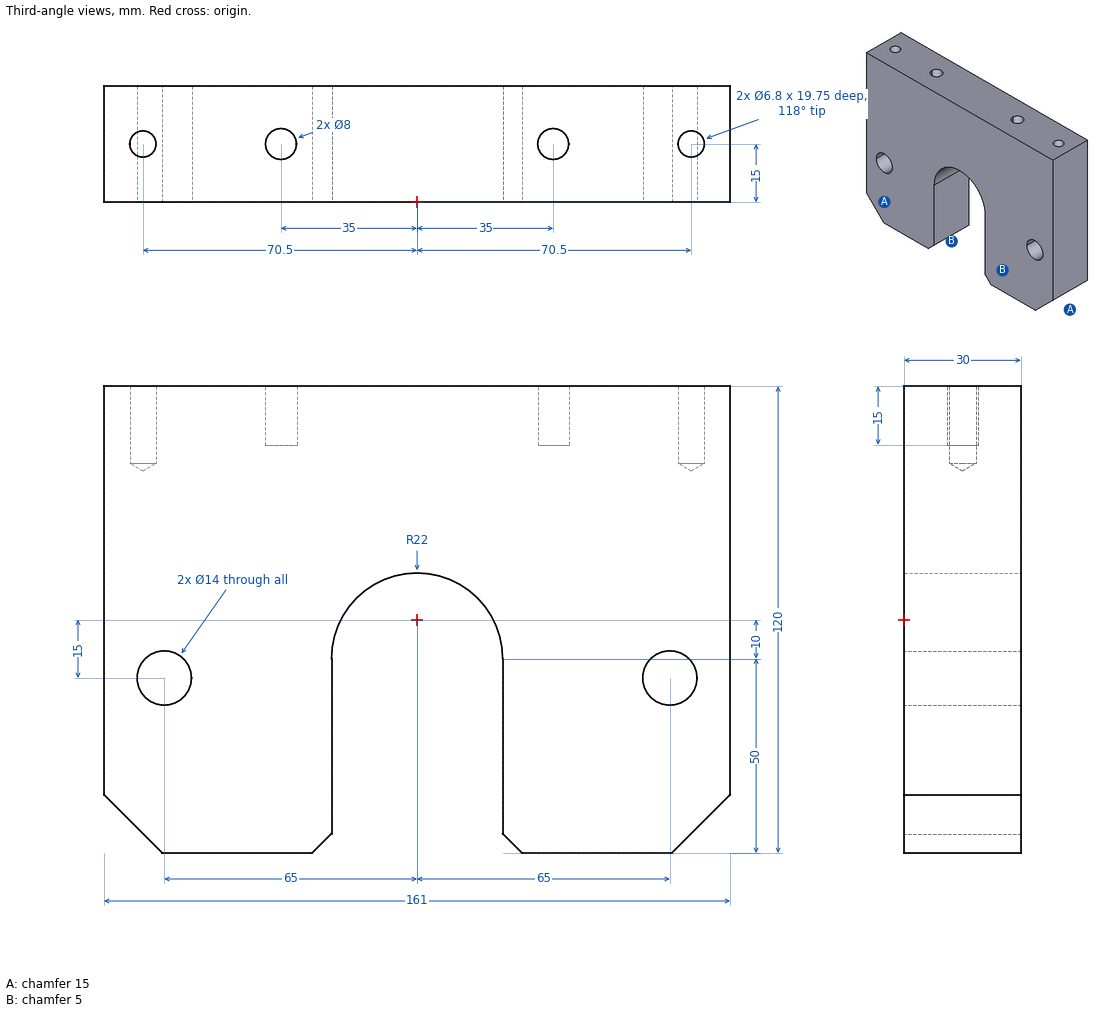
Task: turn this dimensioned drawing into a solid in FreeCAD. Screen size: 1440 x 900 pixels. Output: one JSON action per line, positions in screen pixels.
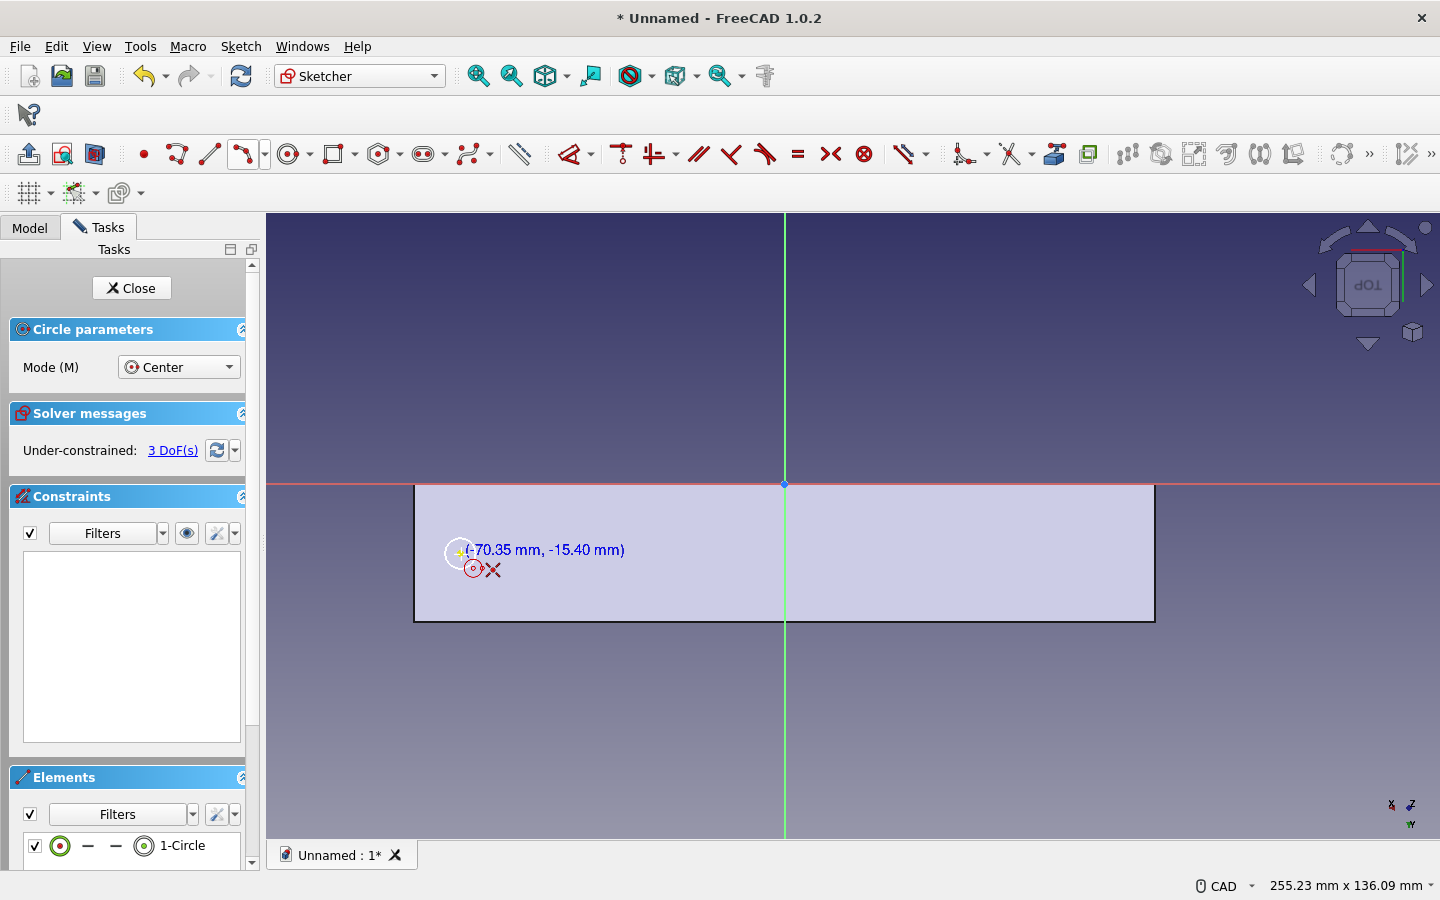
{"action": "scroll", "coordinate": [1109, 553], "scroll_direction": "up", "scroll_amount": 2}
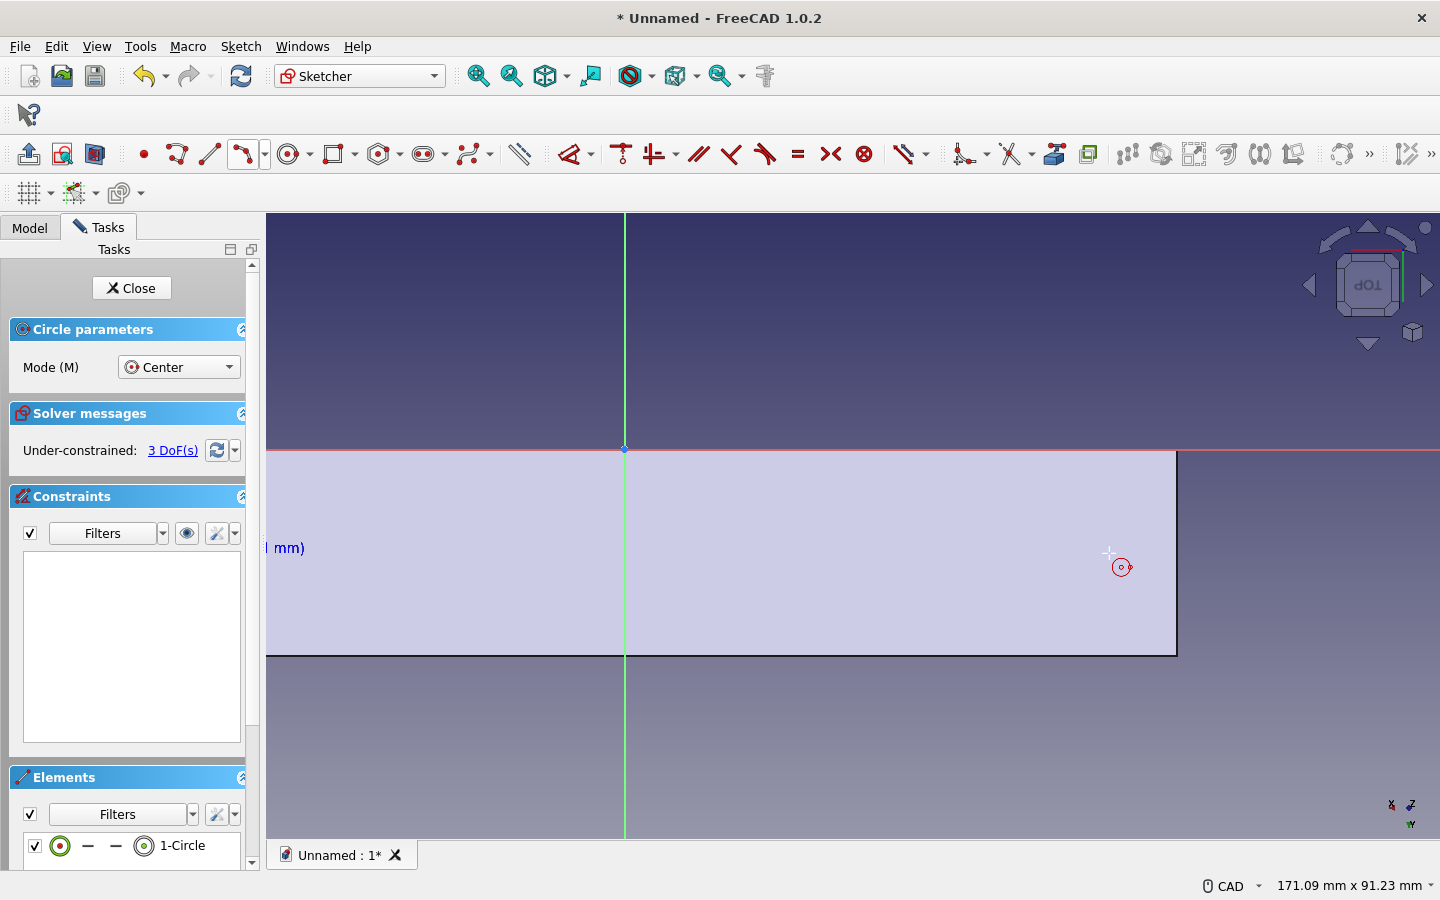
{"action": "left_click", "coordinate": [1109, 553]}
{"action": "left_click", "coordinate": [1125, 536]}
{"action": "key", "text": "Escape"}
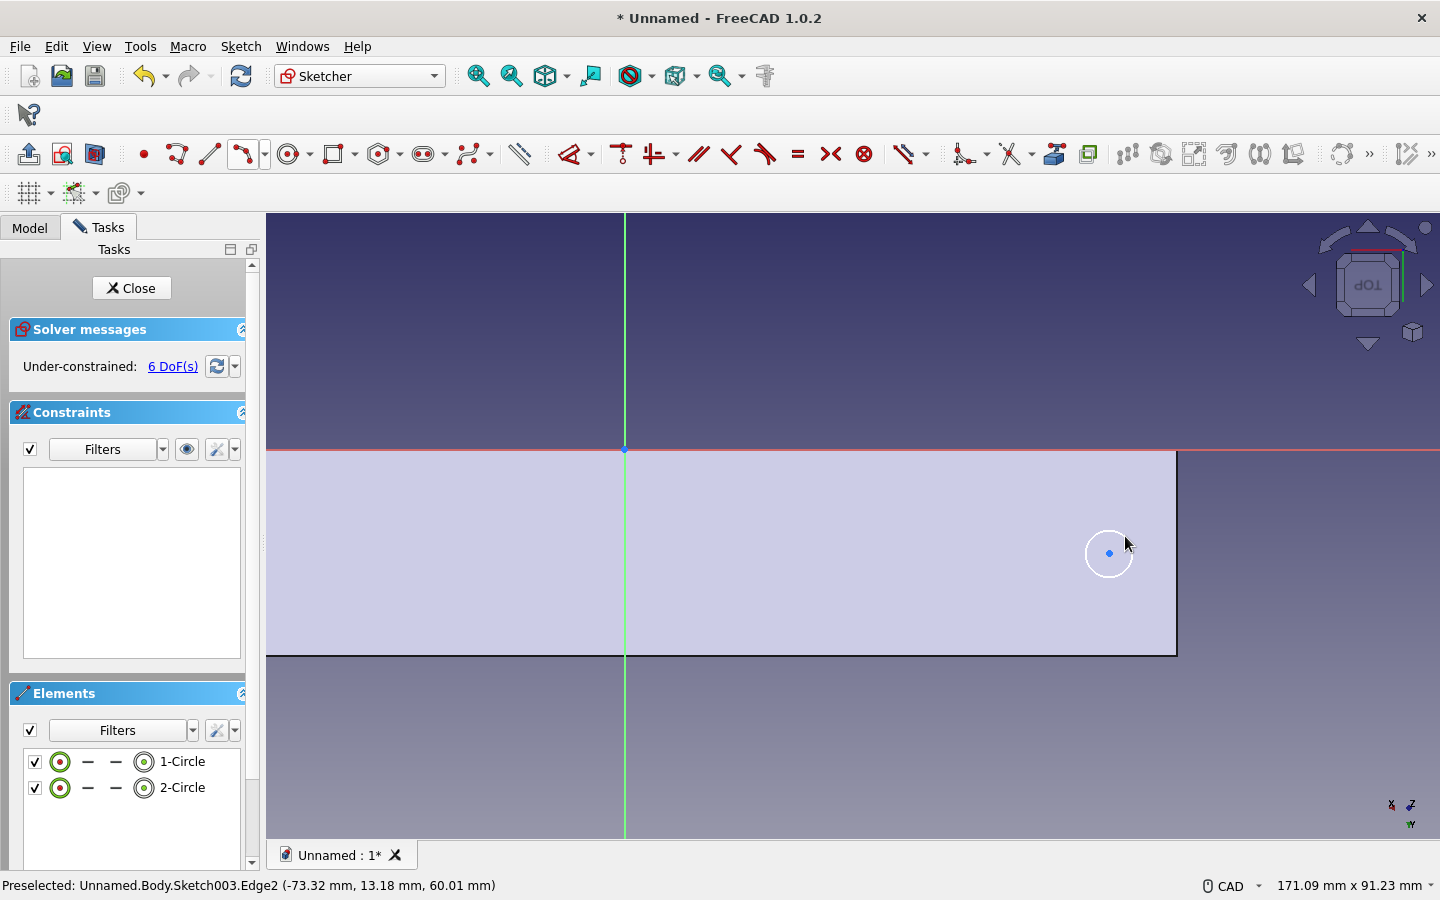
{"action": "scroll", "coordinate": [1109, 553], "scroll_direction": "down", "scroll_amount": 2}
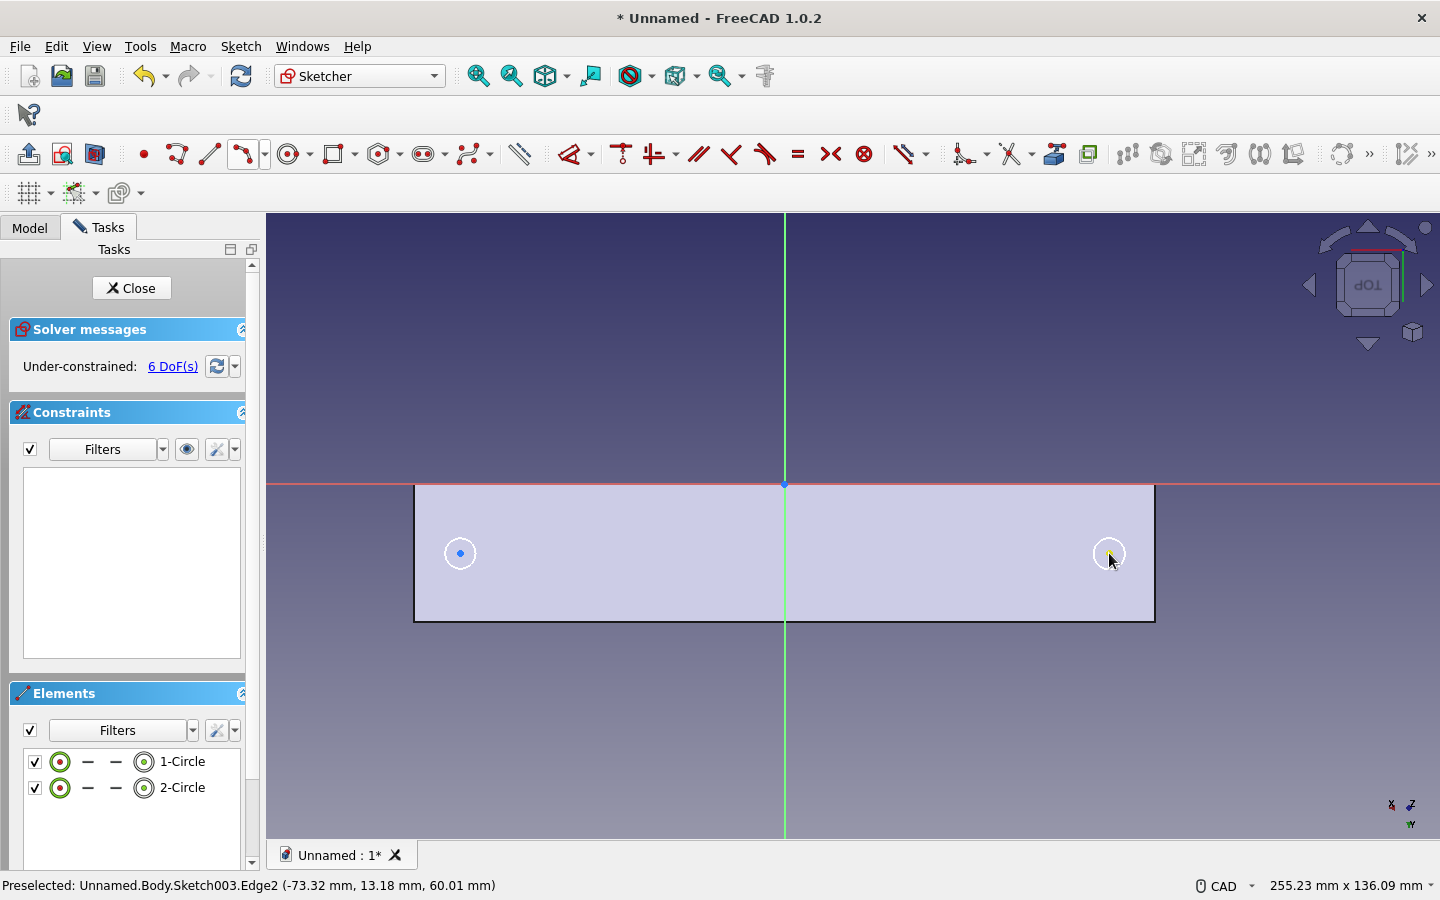
{"action": "left_click", "coordinate": [471, 543]}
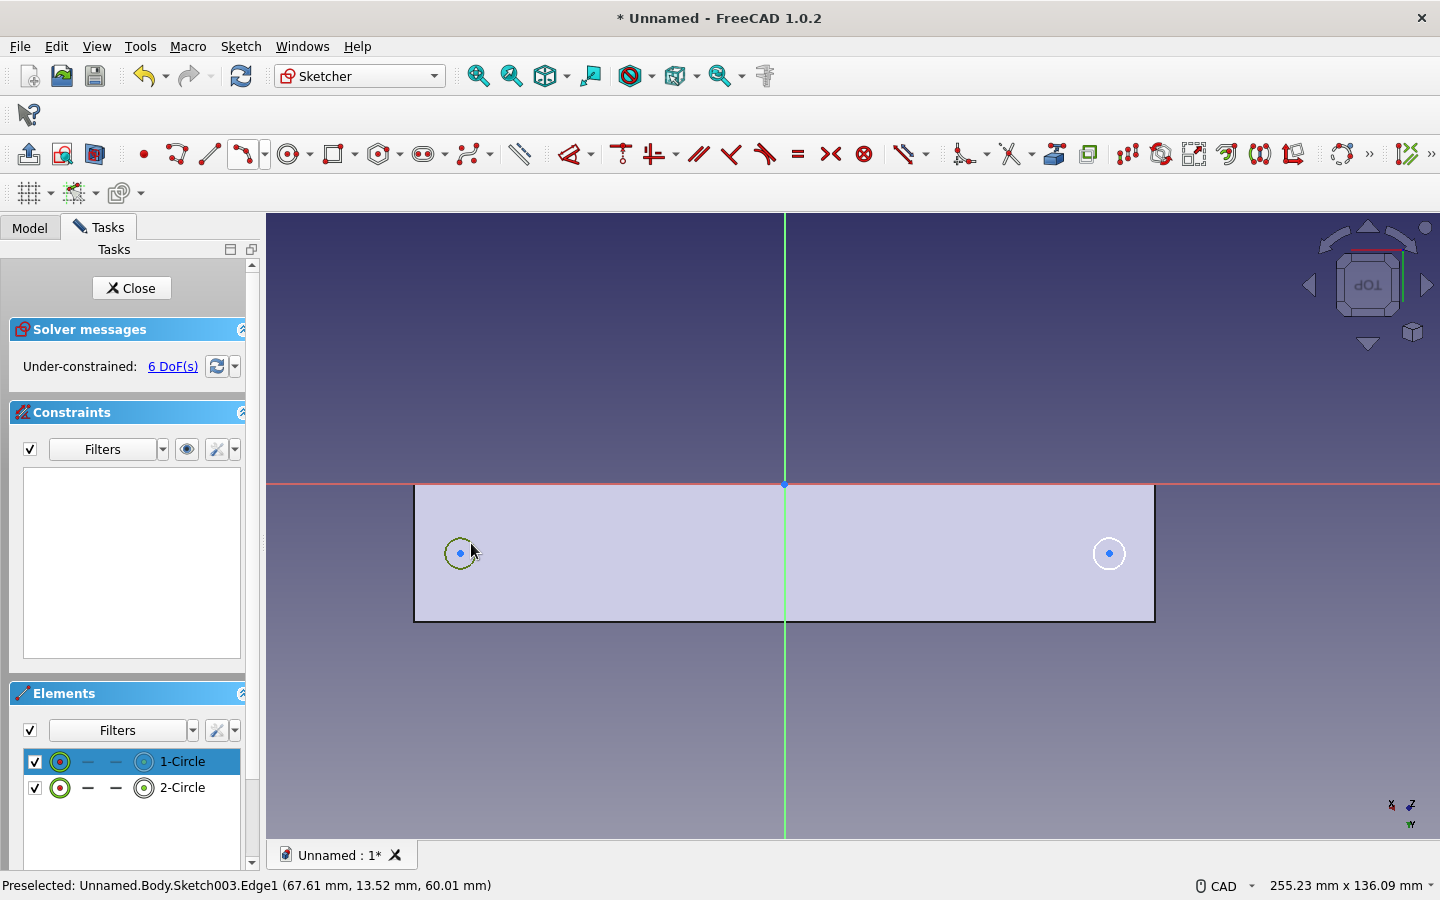
{"action": "left_click", "coordinate": [1120, 543]}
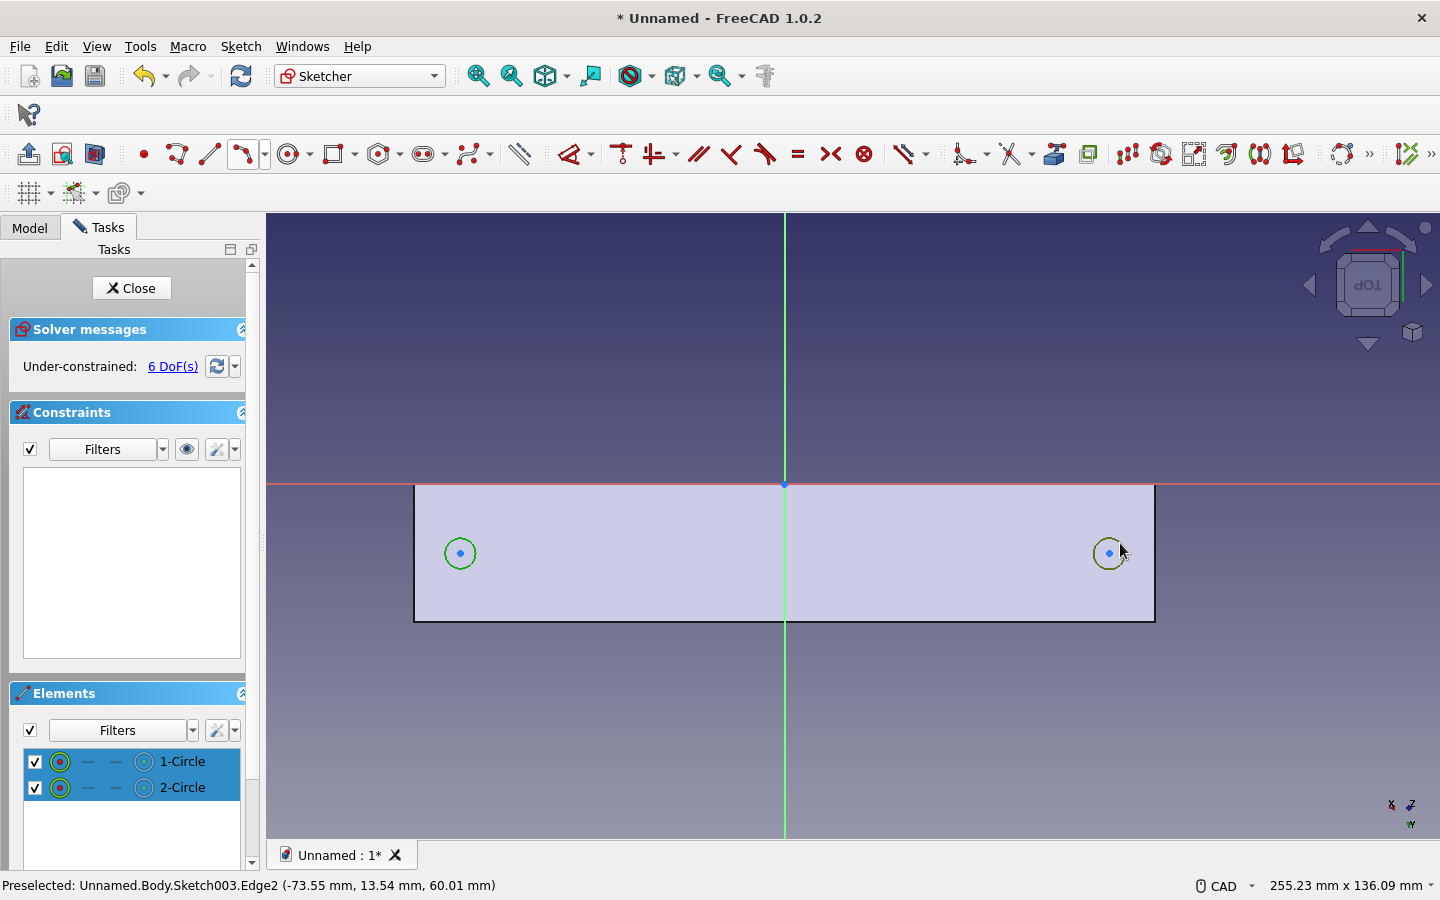
{"action": "left_click", "coordinate": [798, 154]}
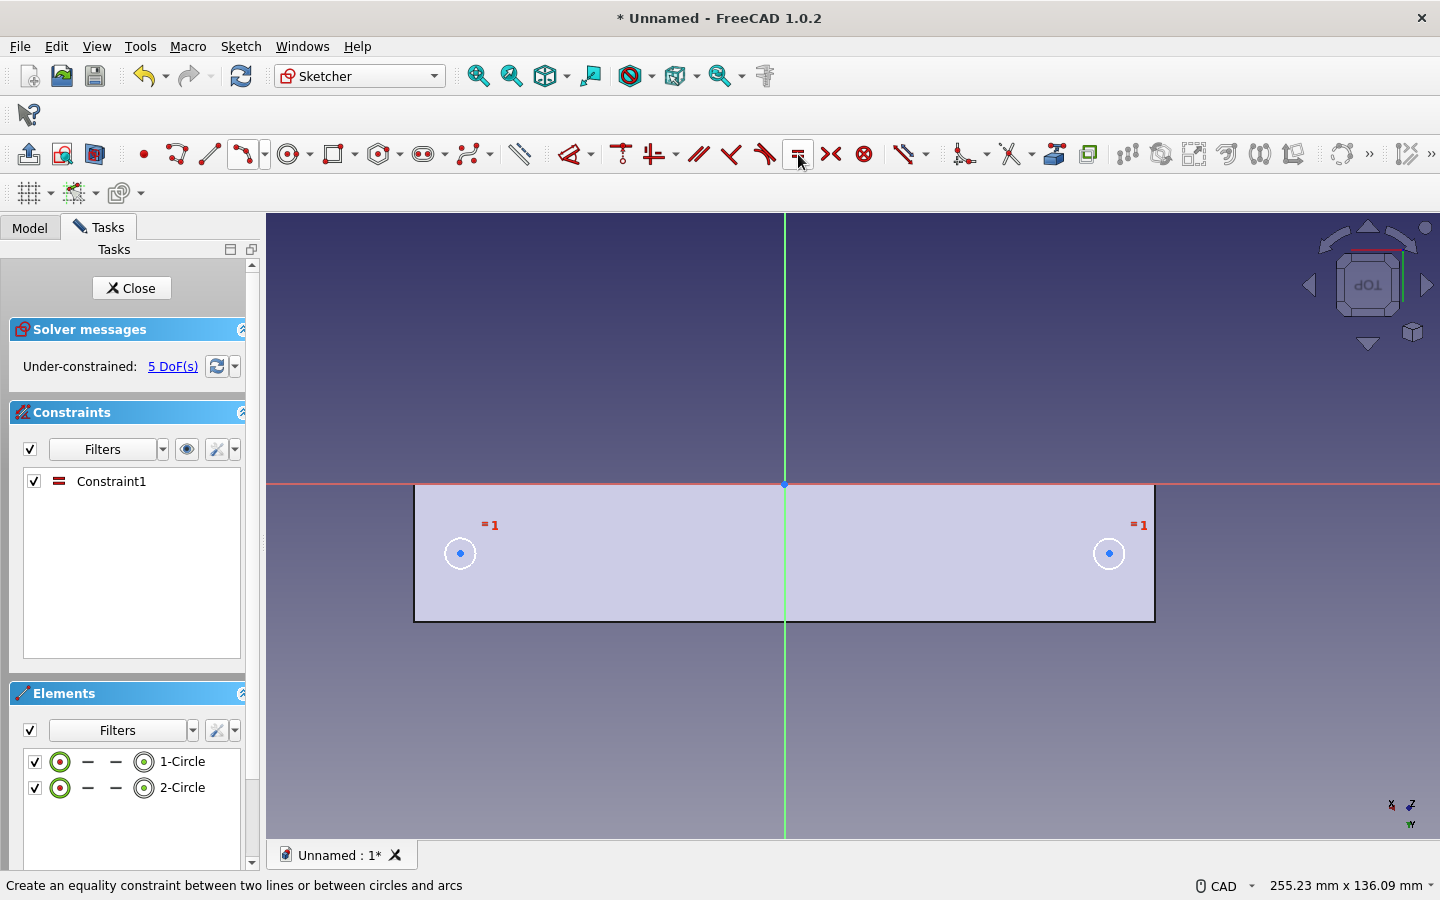
{"action": "left_click", "coordinate": [460, 554]}